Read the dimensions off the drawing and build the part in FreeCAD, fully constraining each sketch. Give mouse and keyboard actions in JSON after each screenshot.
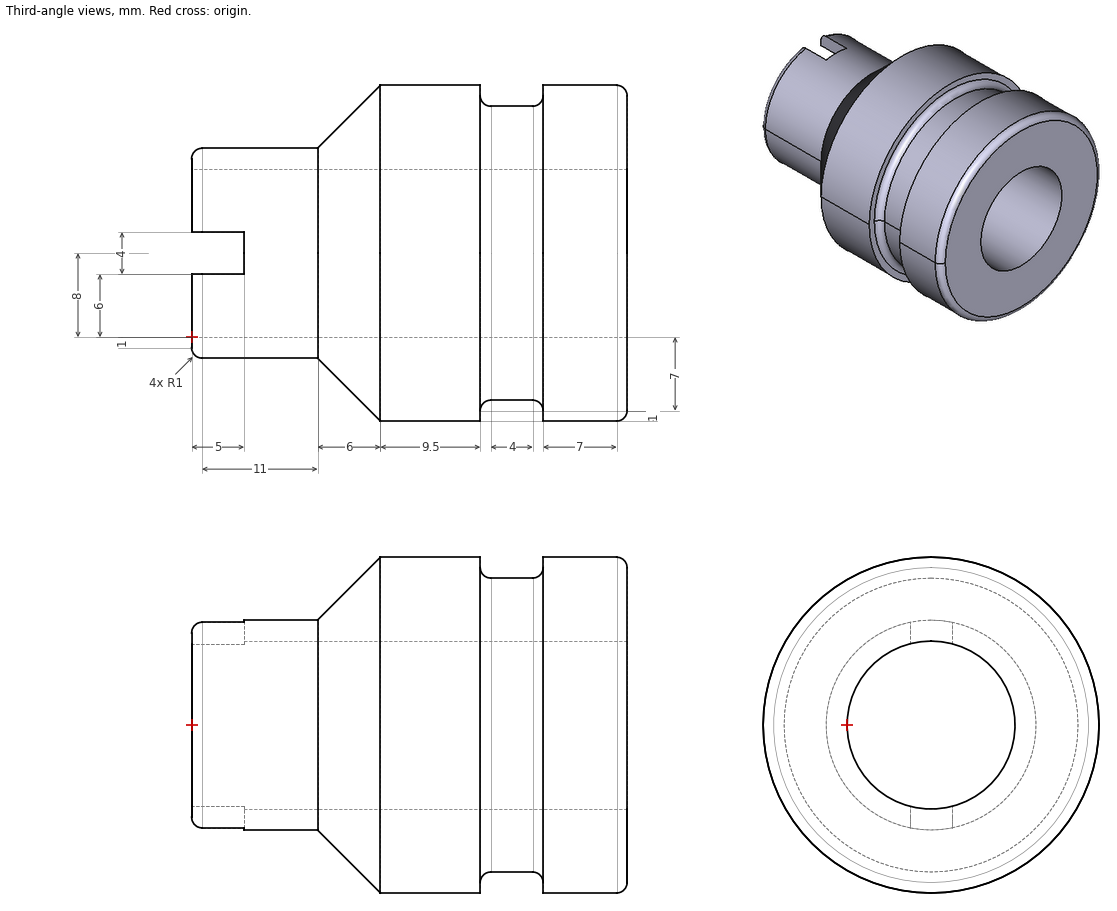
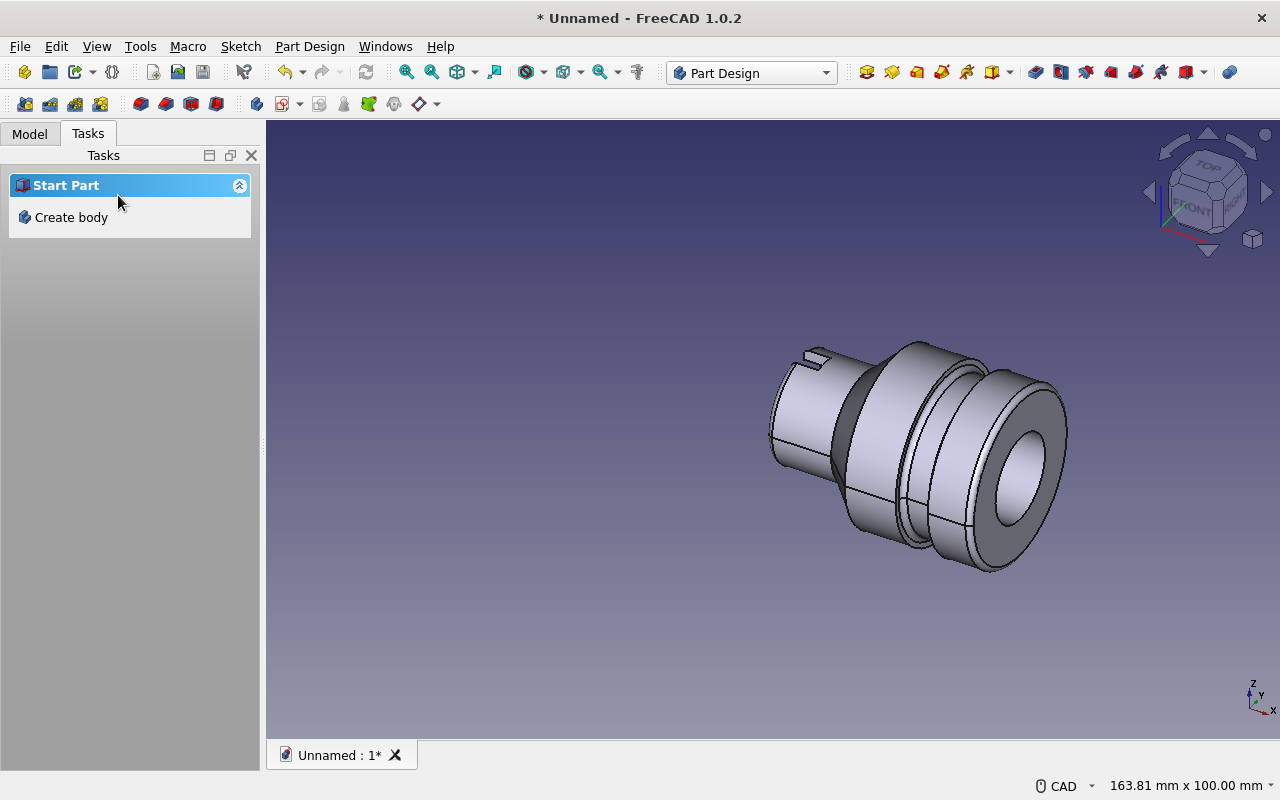
{"action": "key", "text": "0"}